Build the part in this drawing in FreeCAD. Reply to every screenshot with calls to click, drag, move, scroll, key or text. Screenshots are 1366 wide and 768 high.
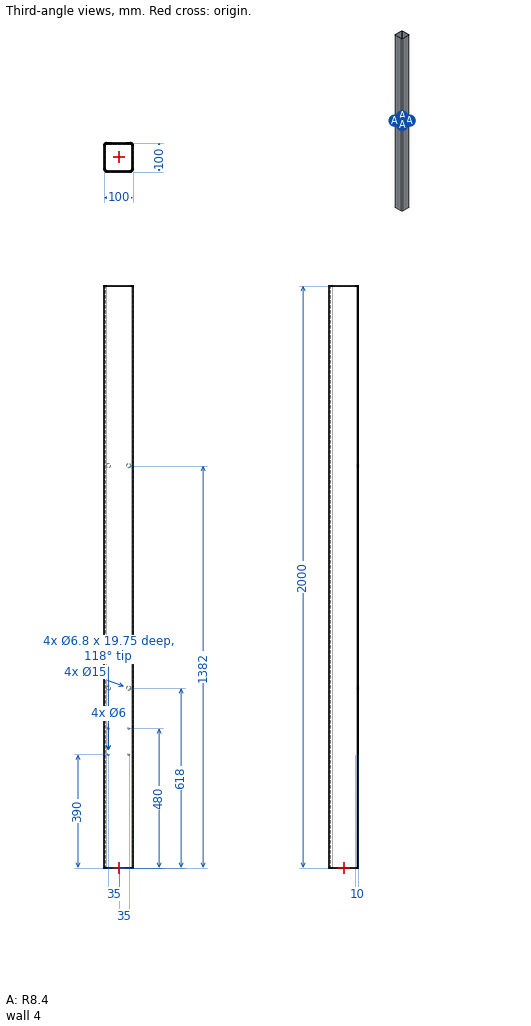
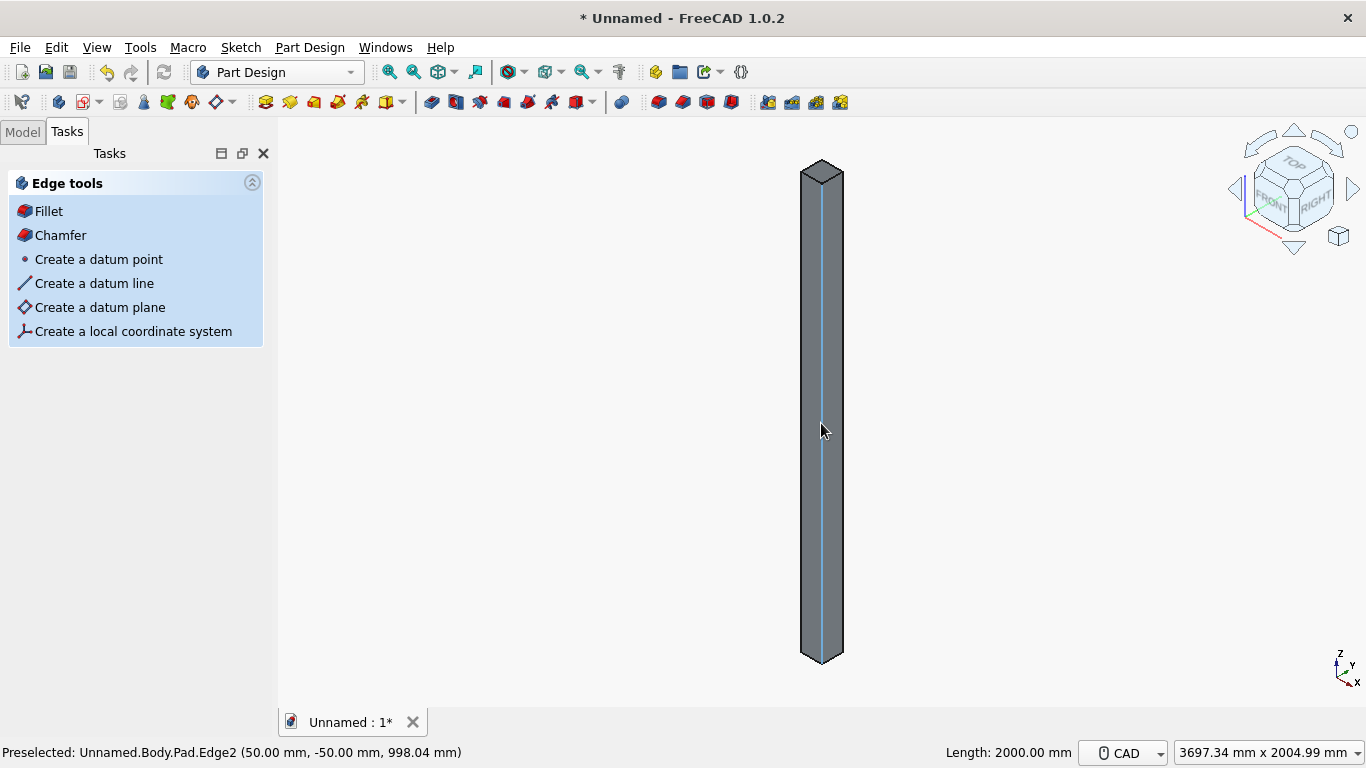
key(2)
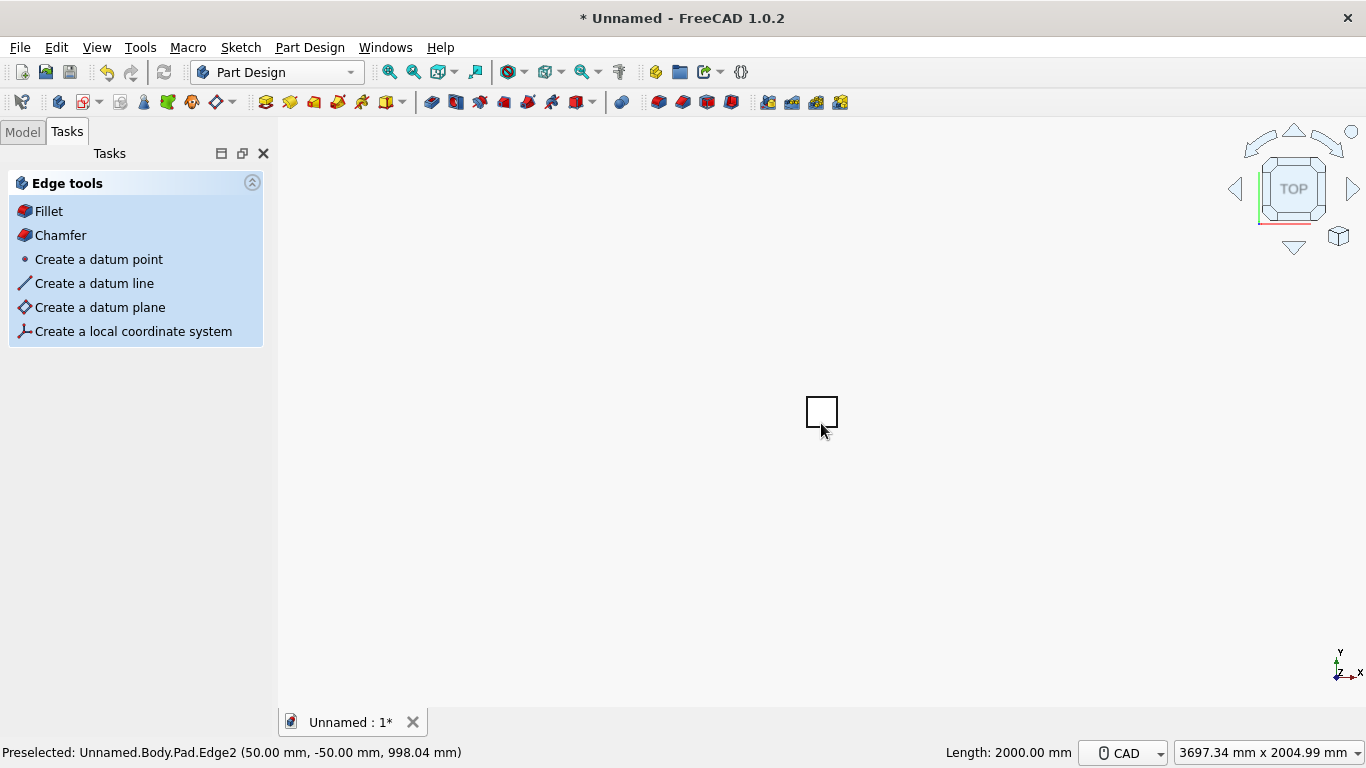
click(390, 72)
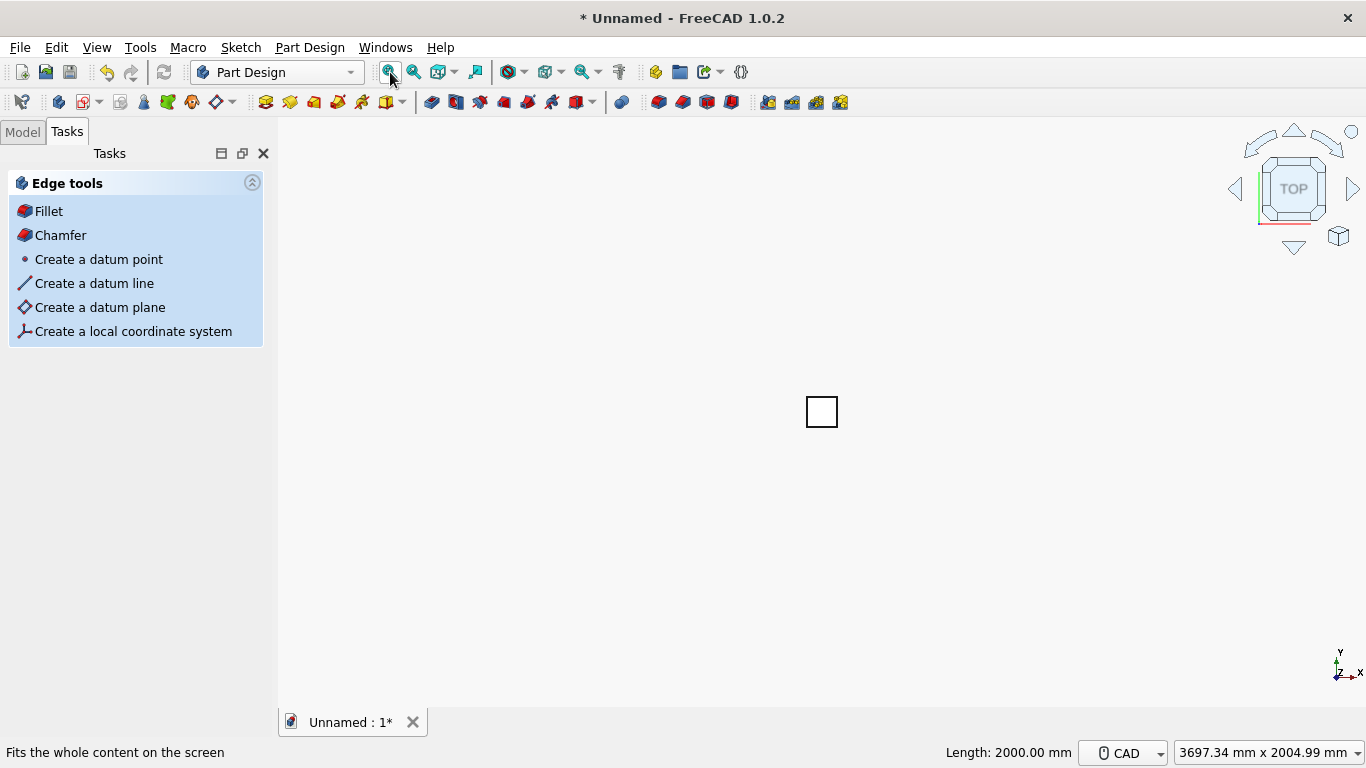
key(1)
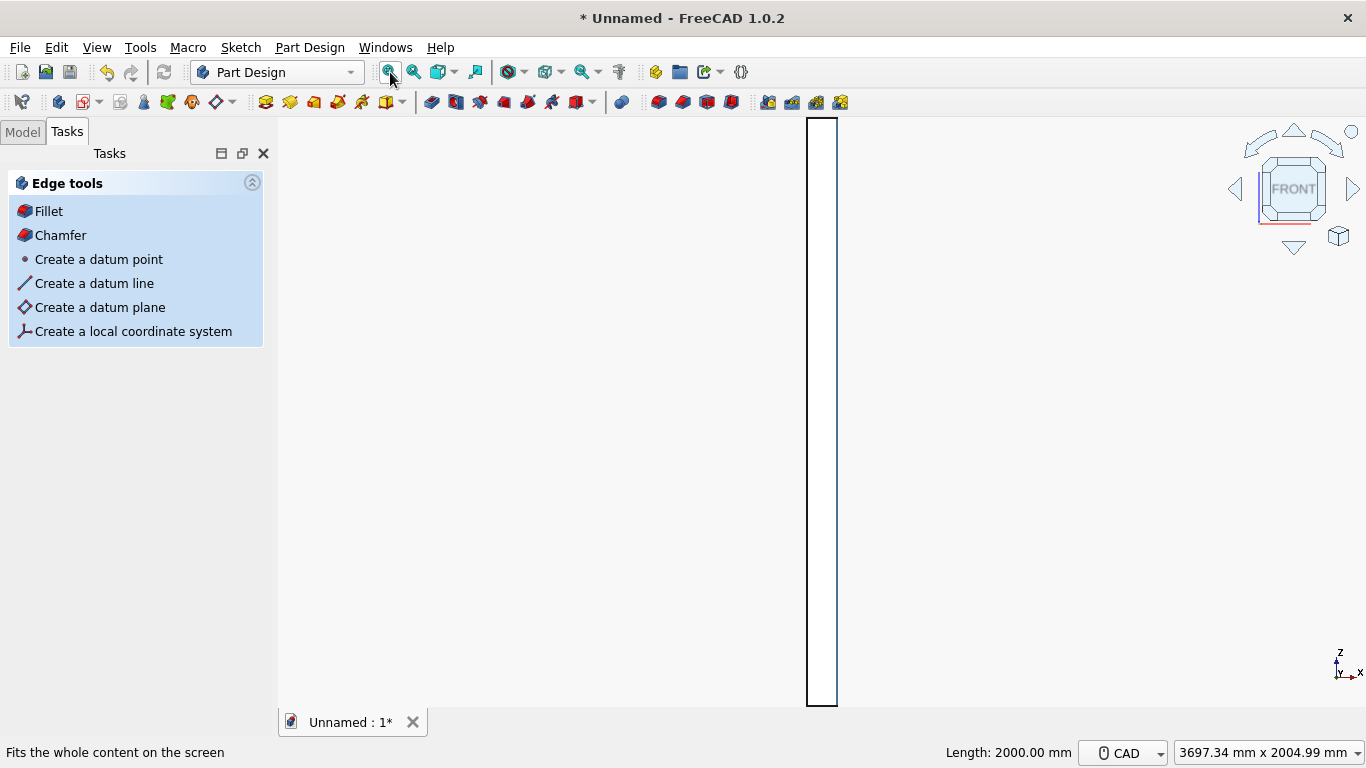
click(807, 411, ctrl)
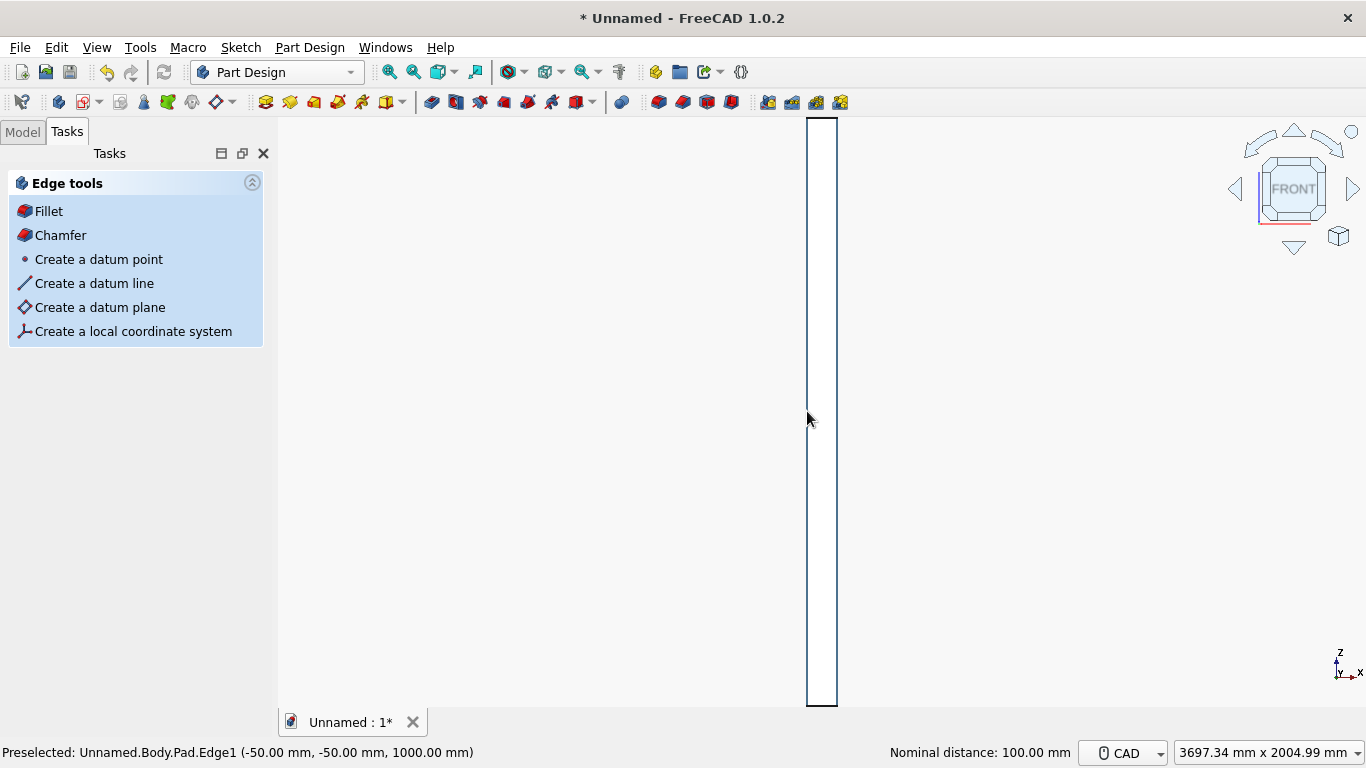
key(3)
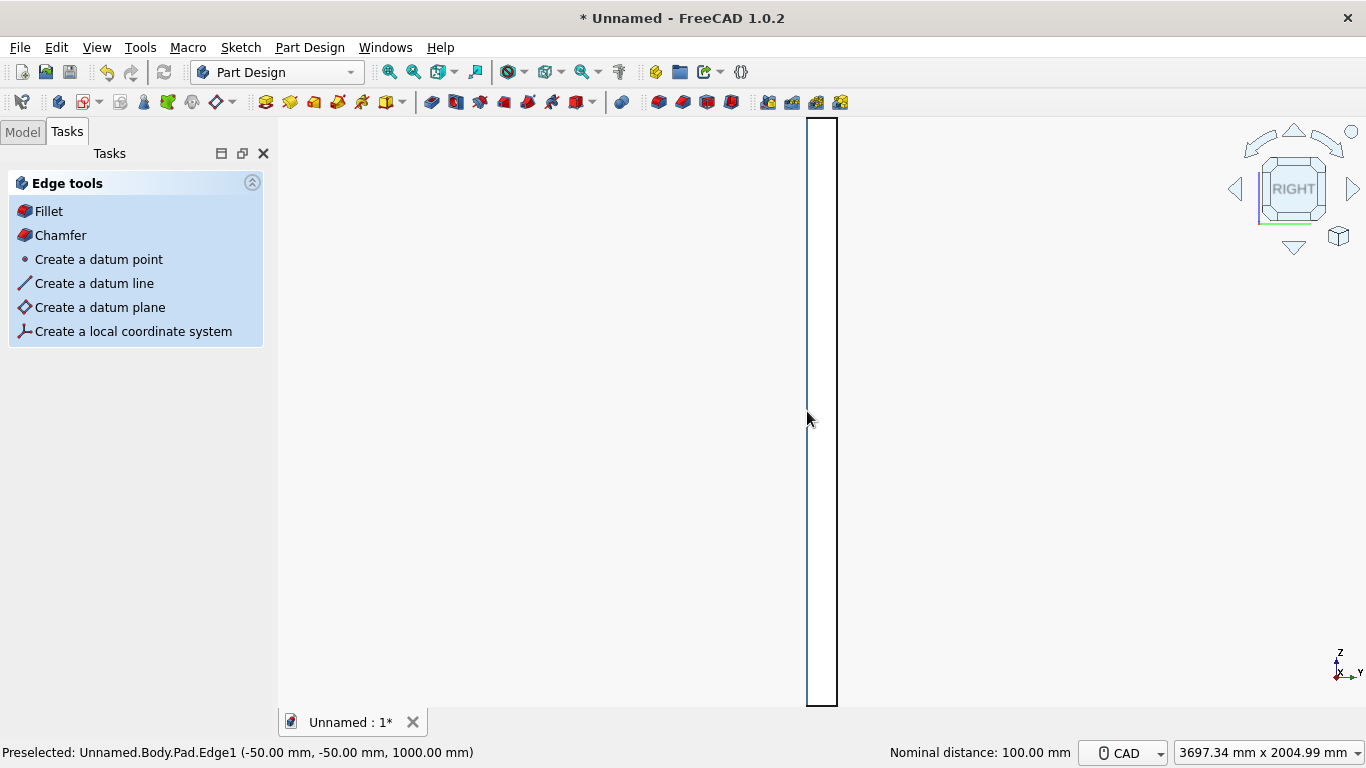
click(837, 411, ctrl)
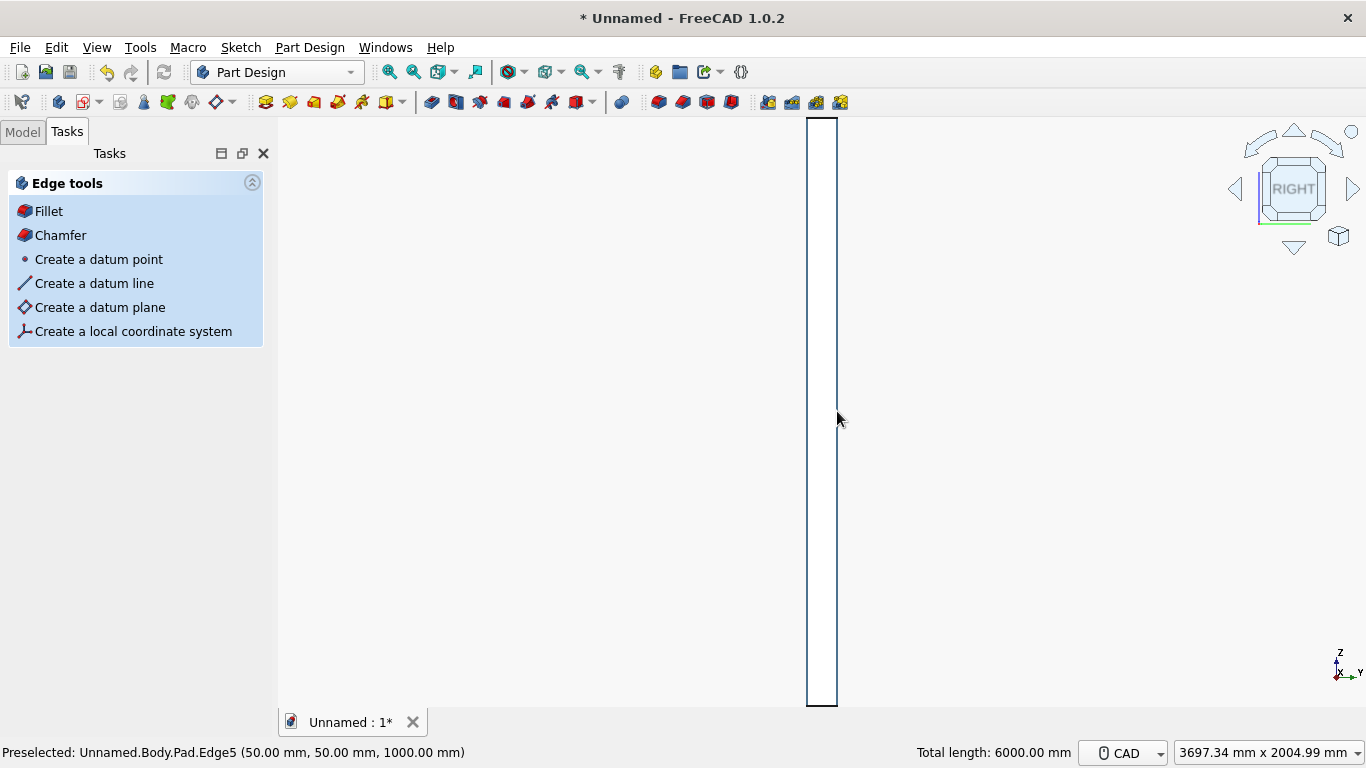
key(5)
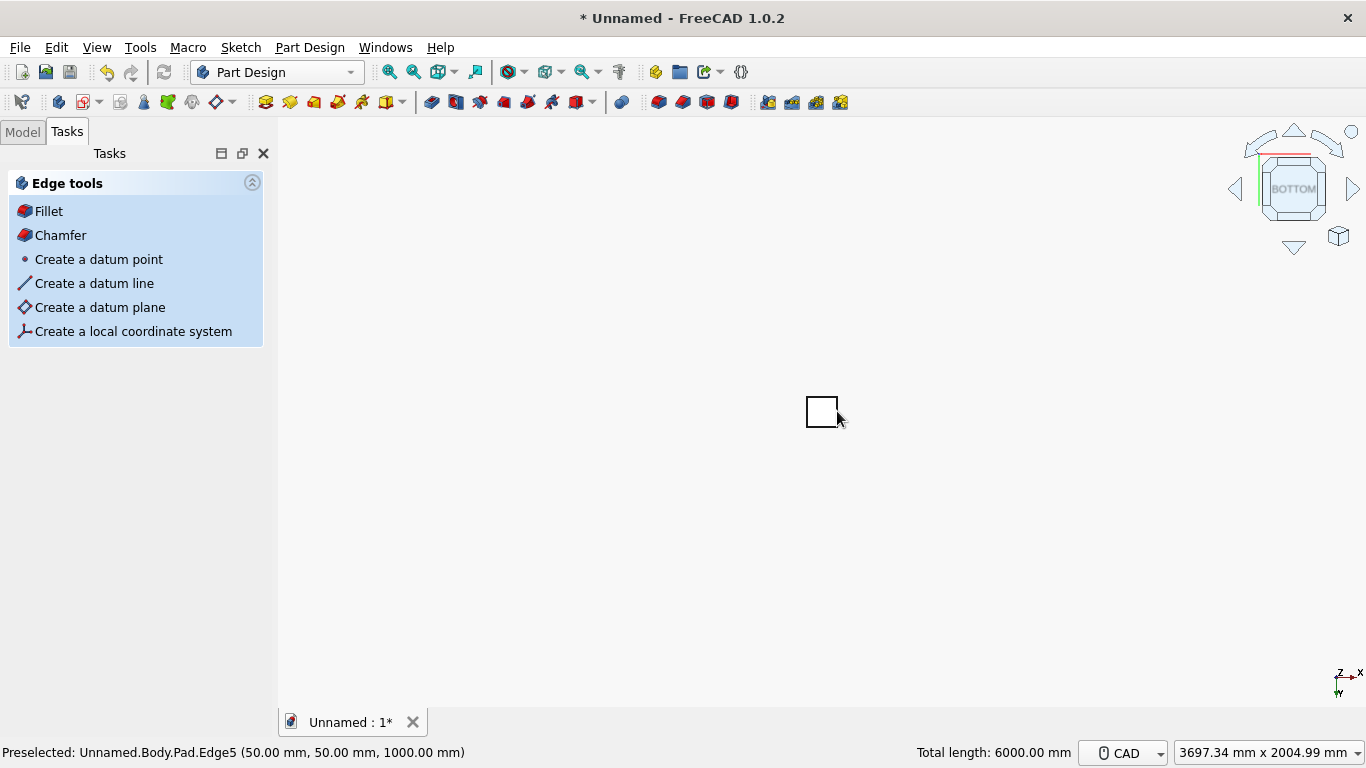
click(390, 72)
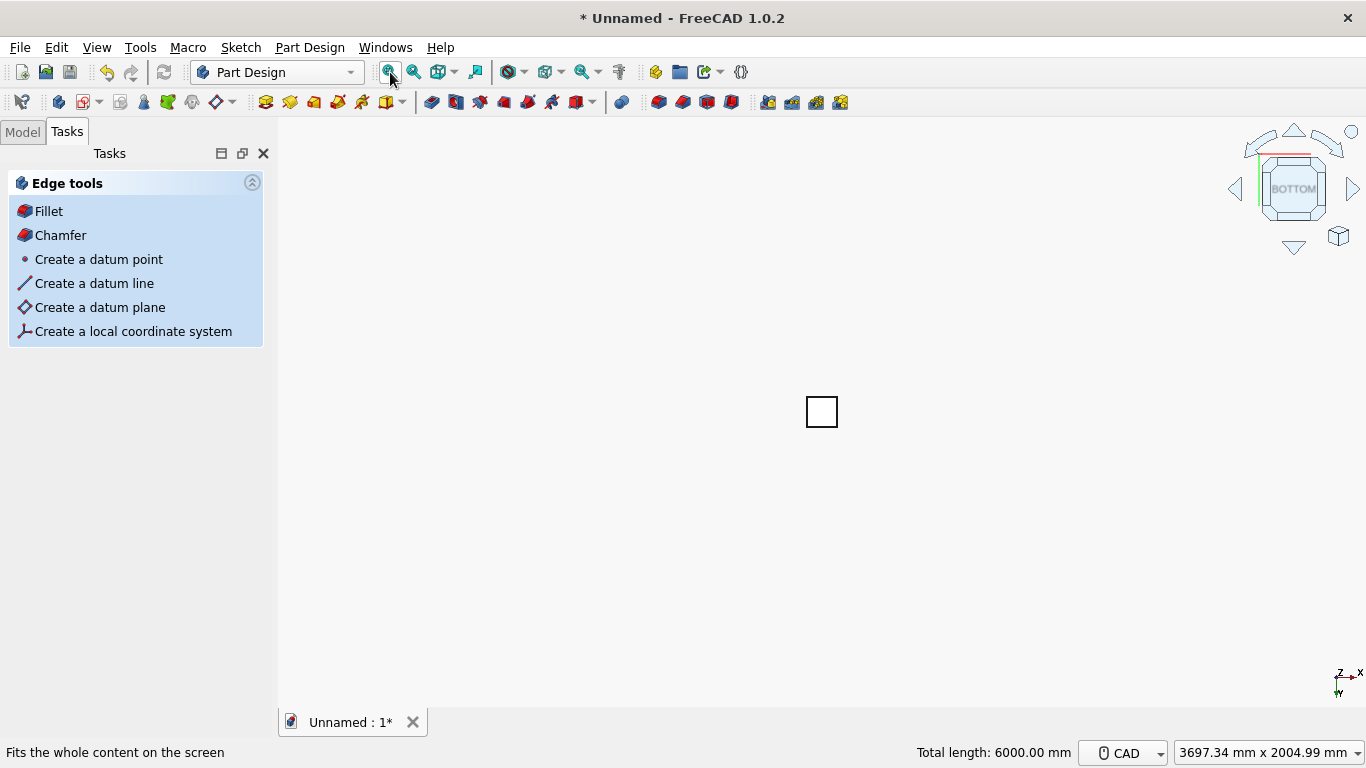
key(4)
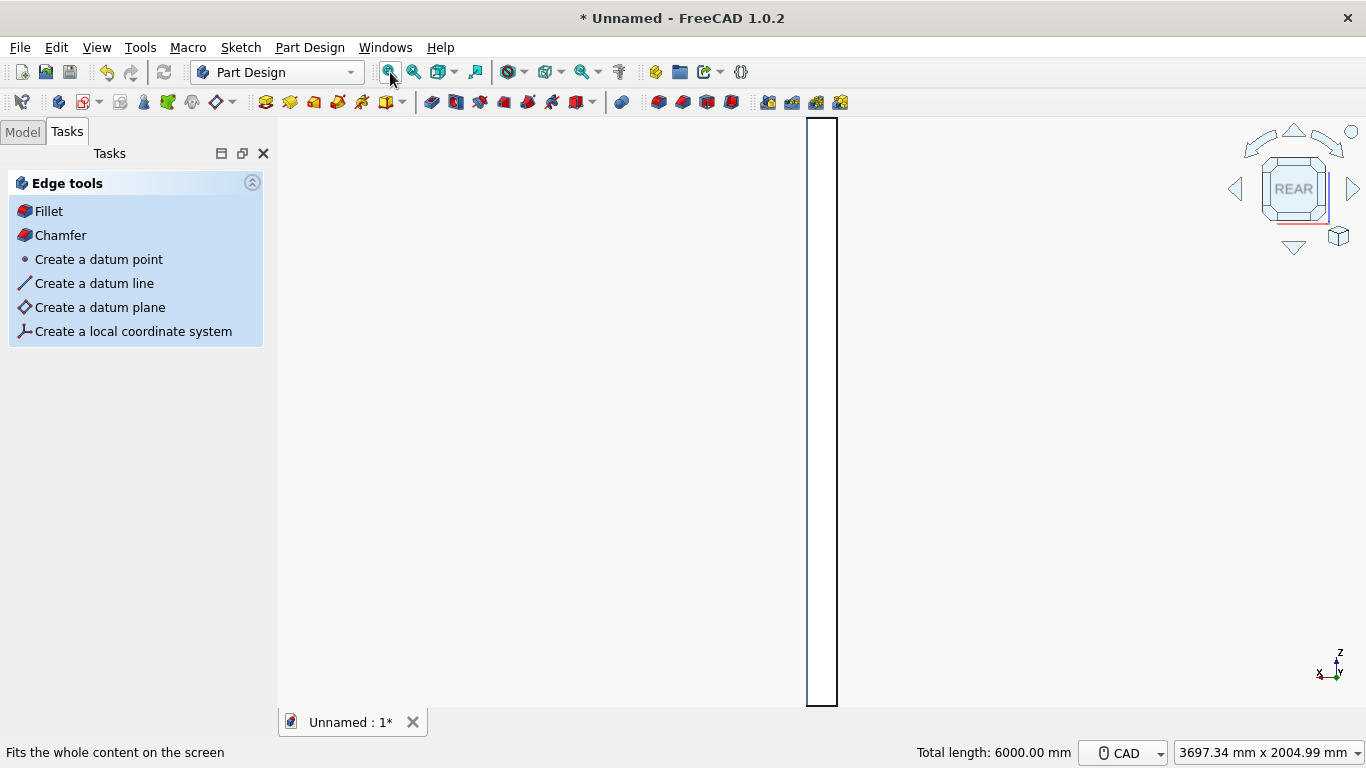
click(837, 411, ctrl)